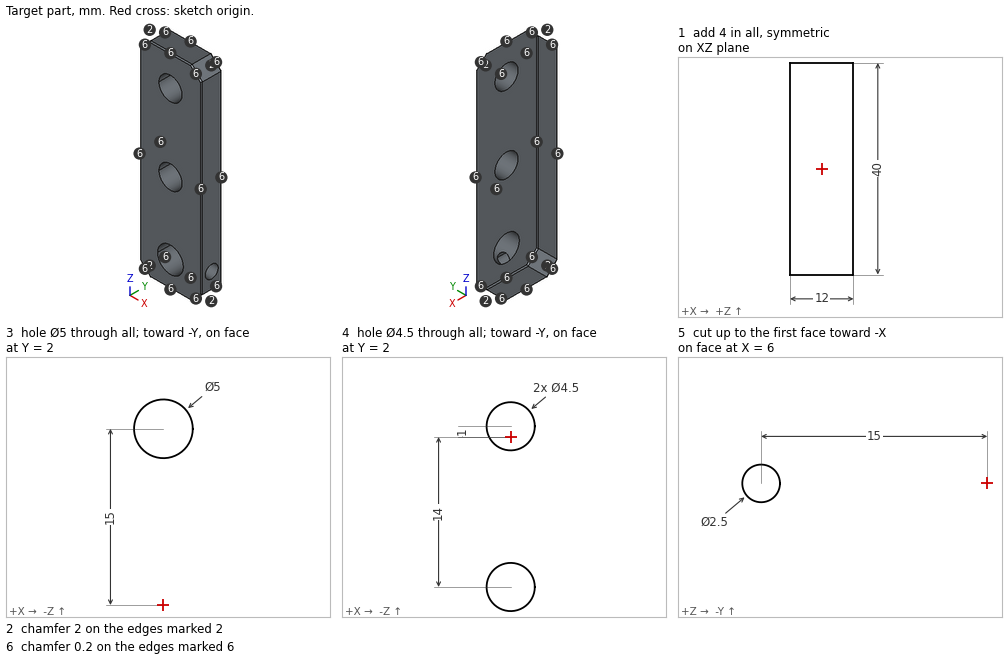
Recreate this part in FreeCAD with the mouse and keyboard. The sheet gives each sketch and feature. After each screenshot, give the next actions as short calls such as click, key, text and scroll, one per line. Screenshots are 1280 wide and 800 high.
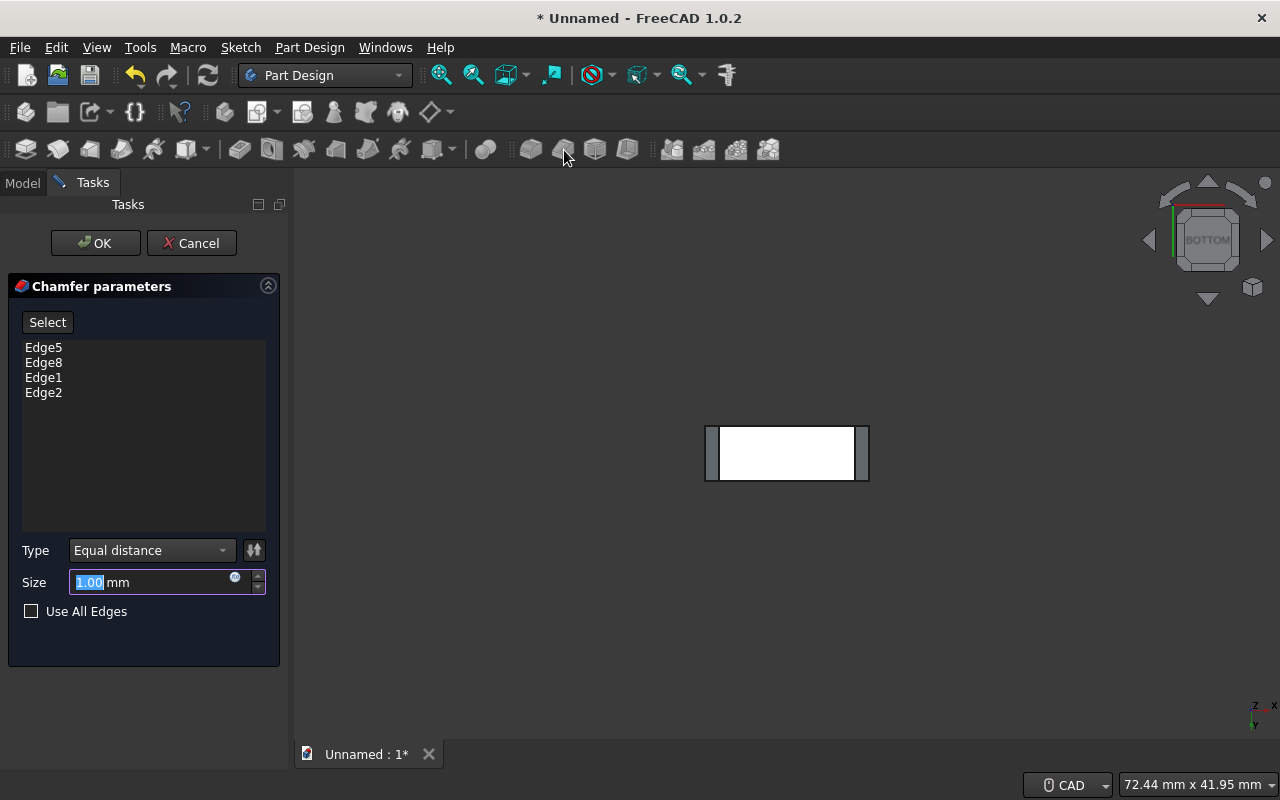
text(2)
key(Tab)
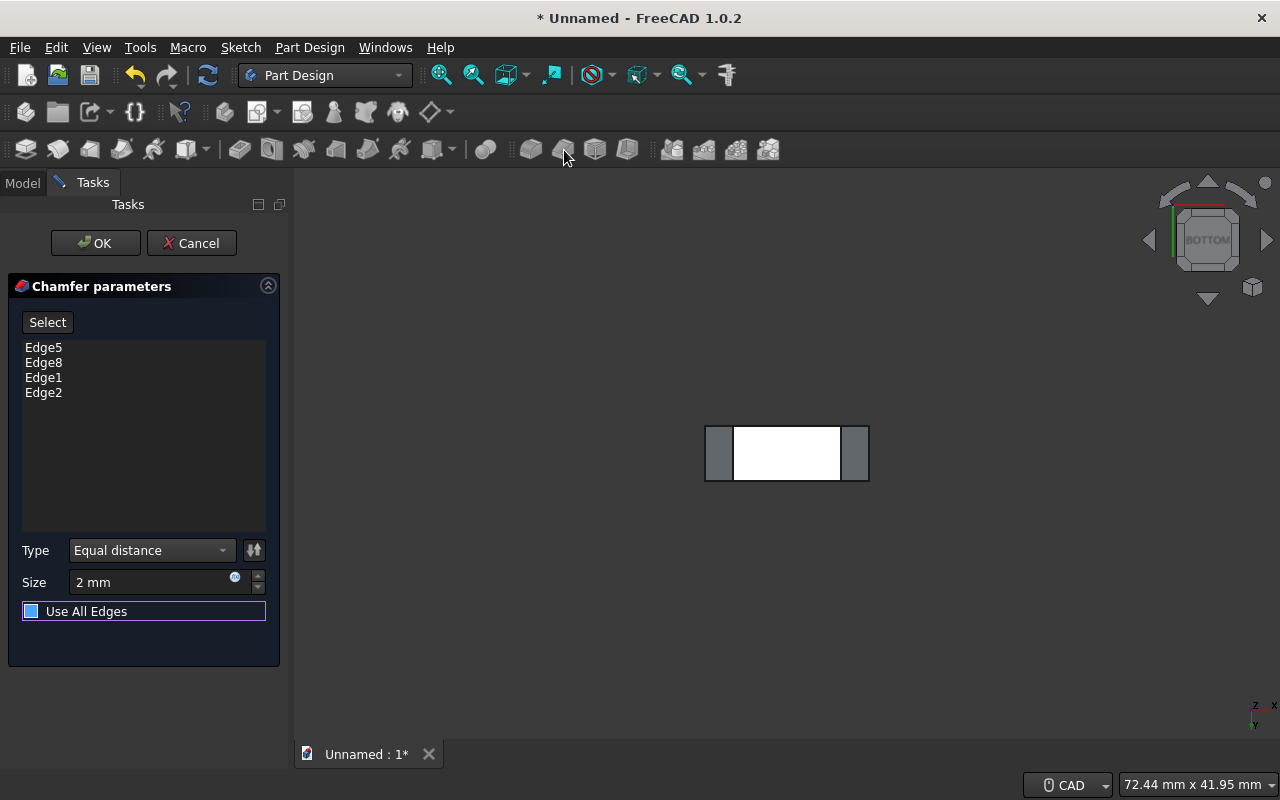
click(96, 243)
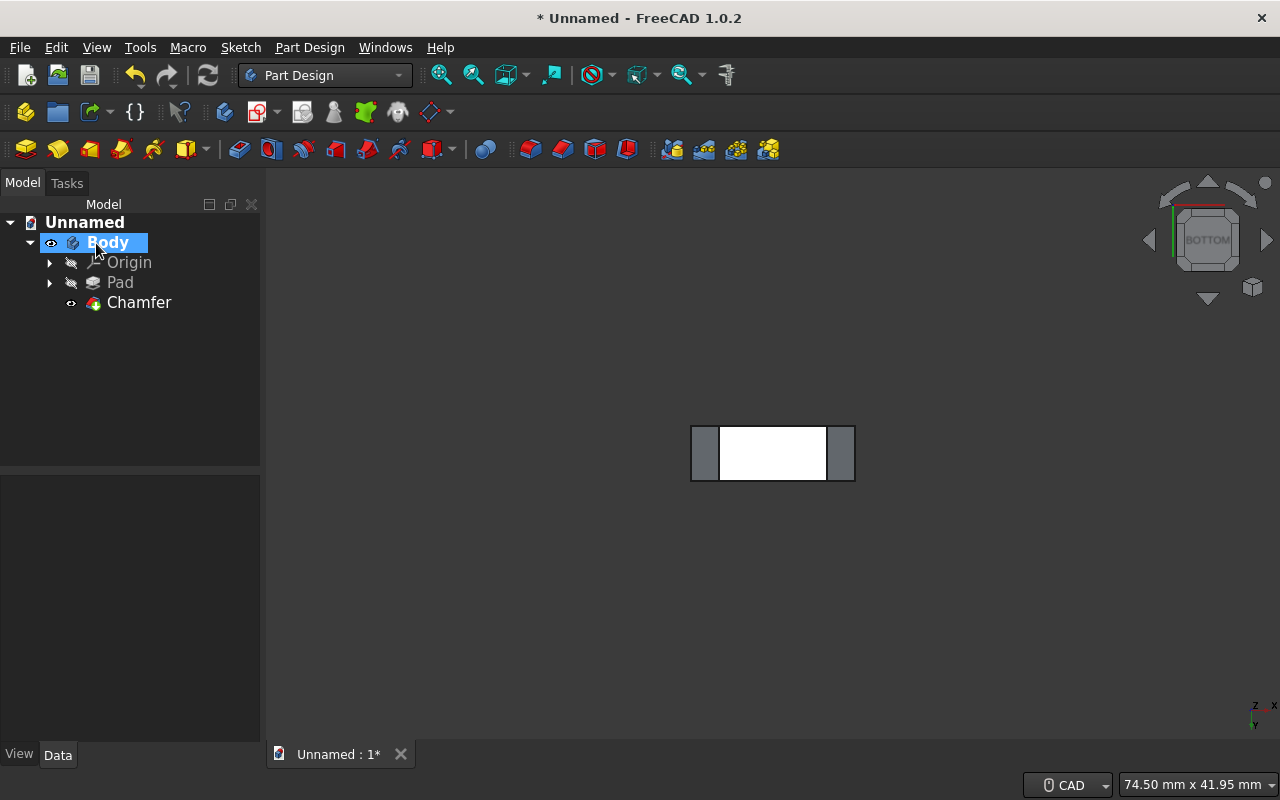
click(442, 76)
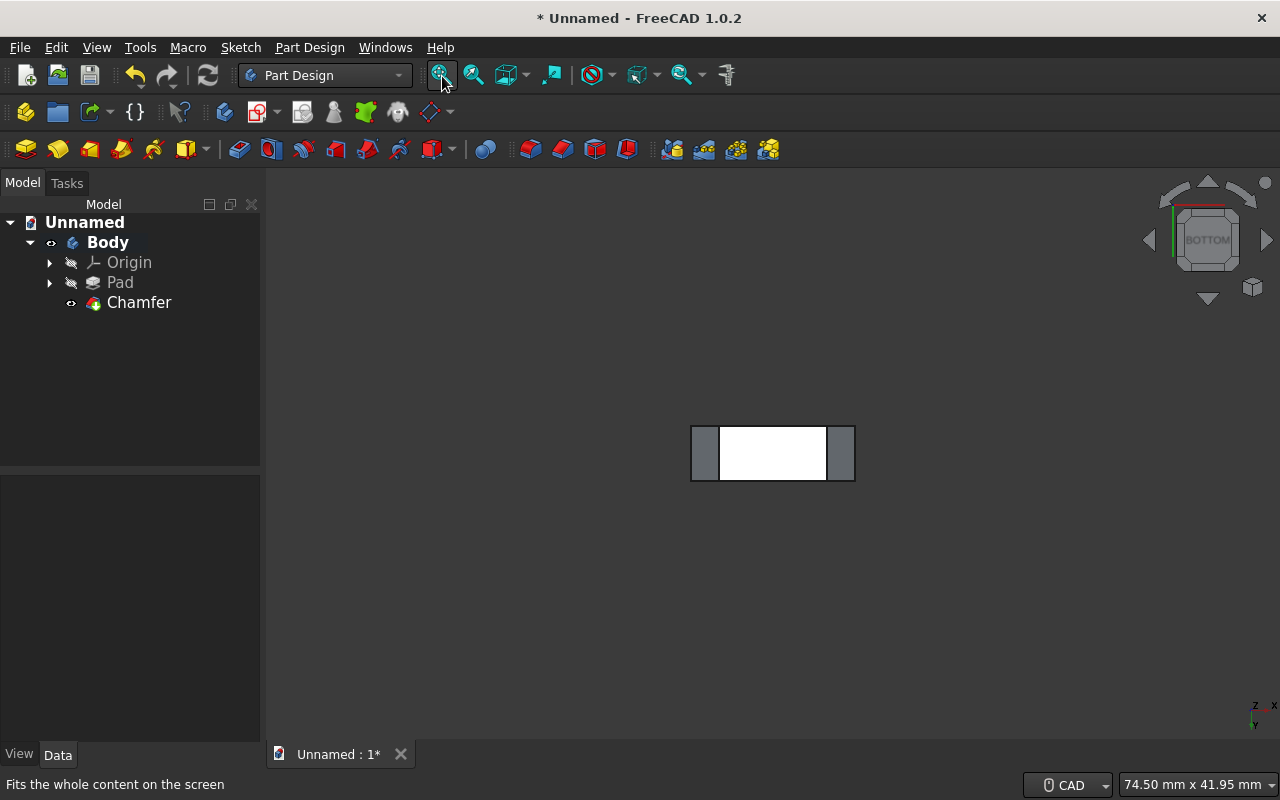
key(4)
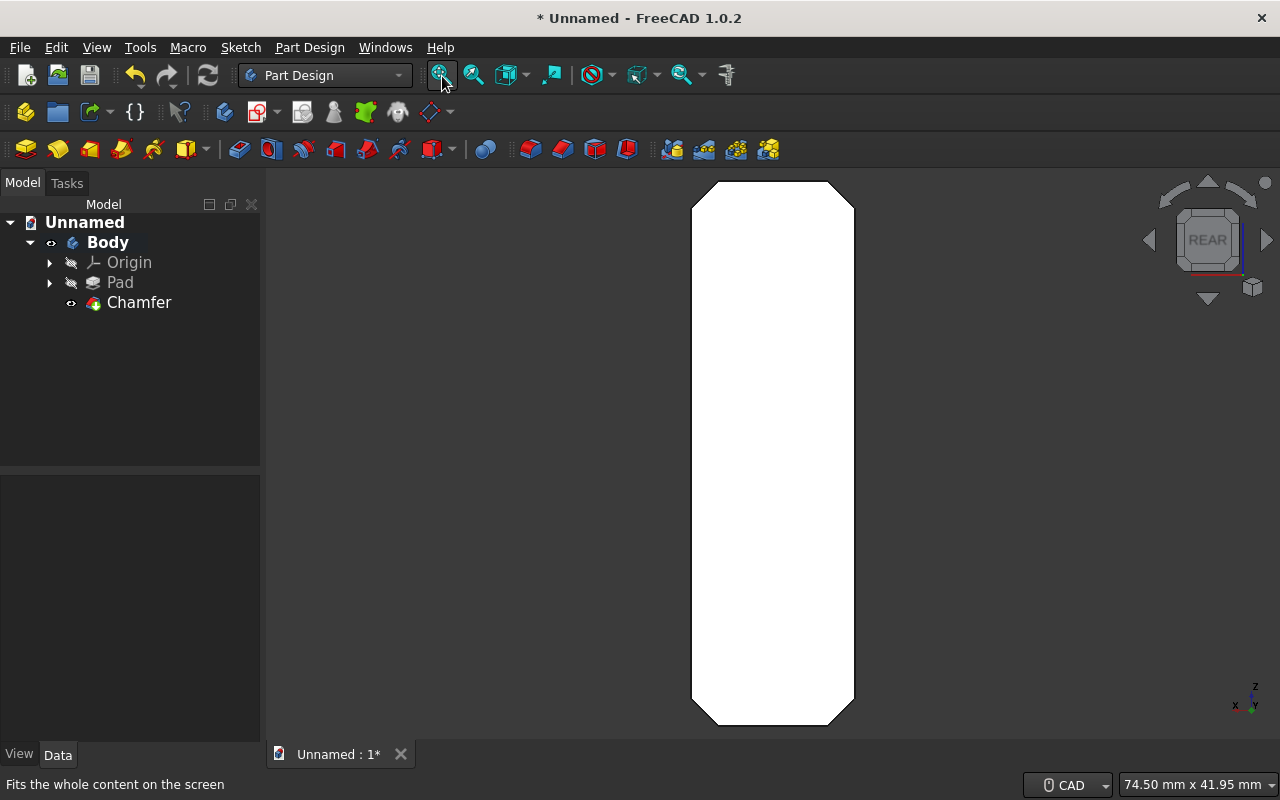
click(773, 297)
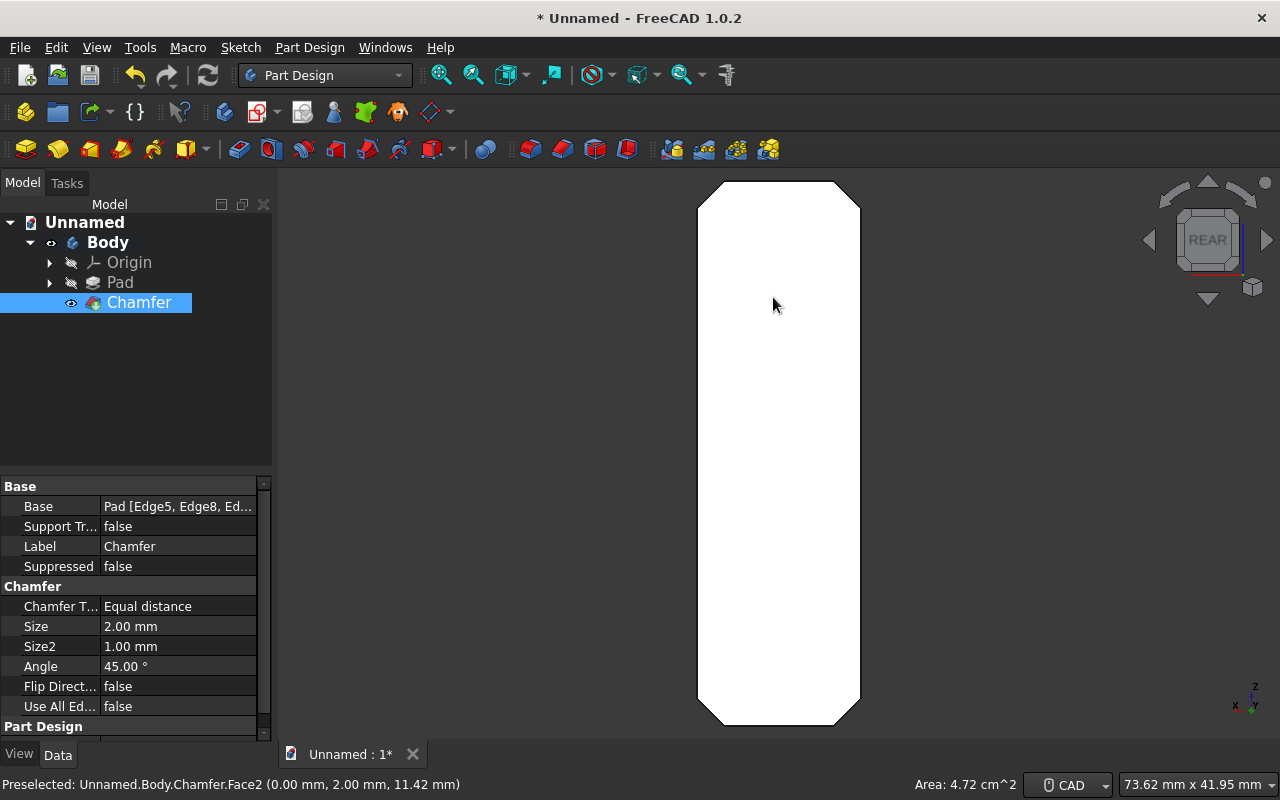
click(258, 112)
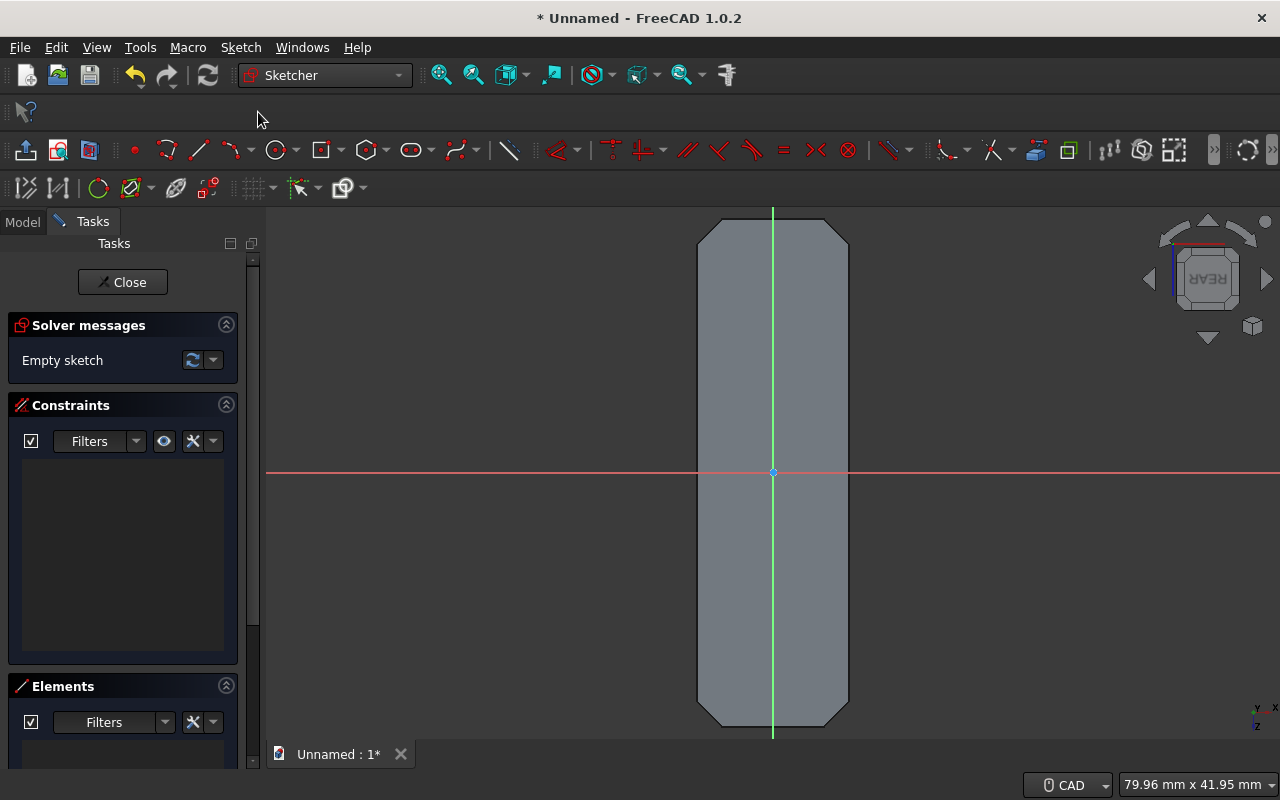
scroll(790, 235, up, 8)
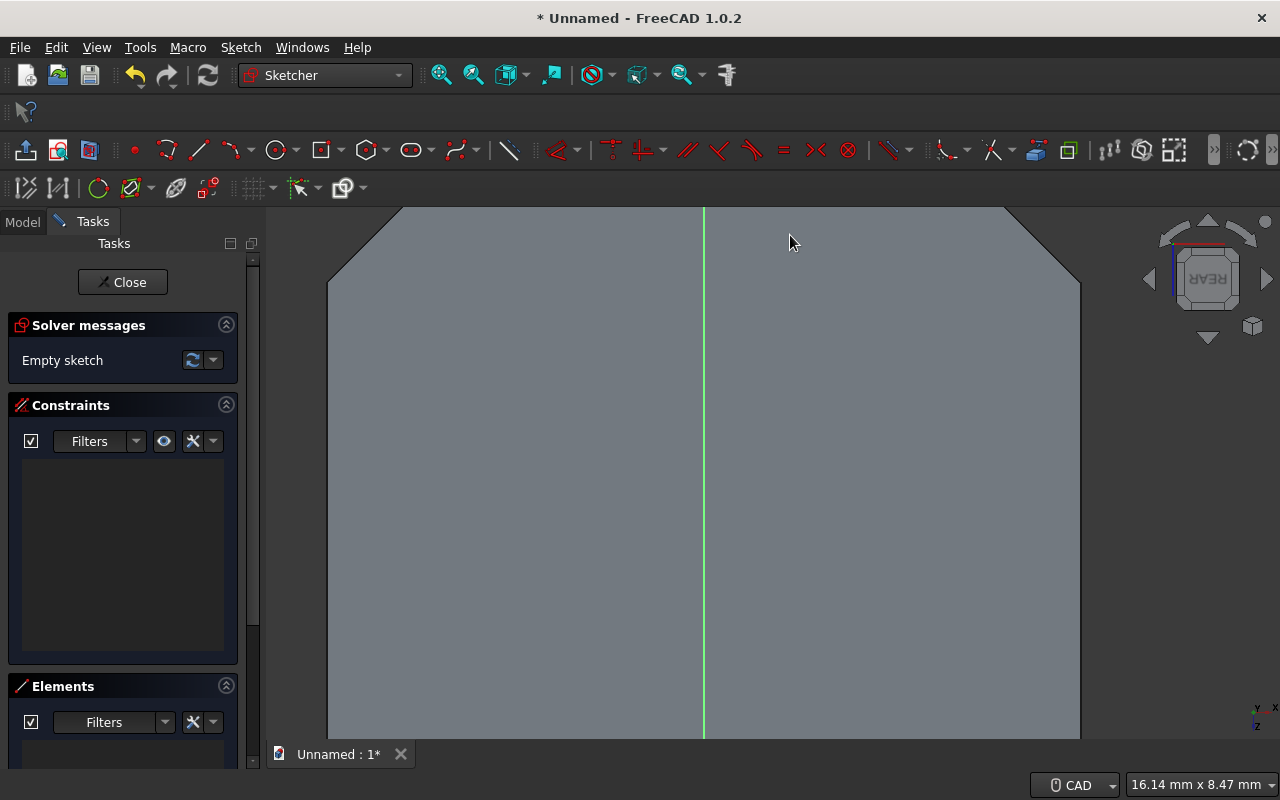
click(276, 150)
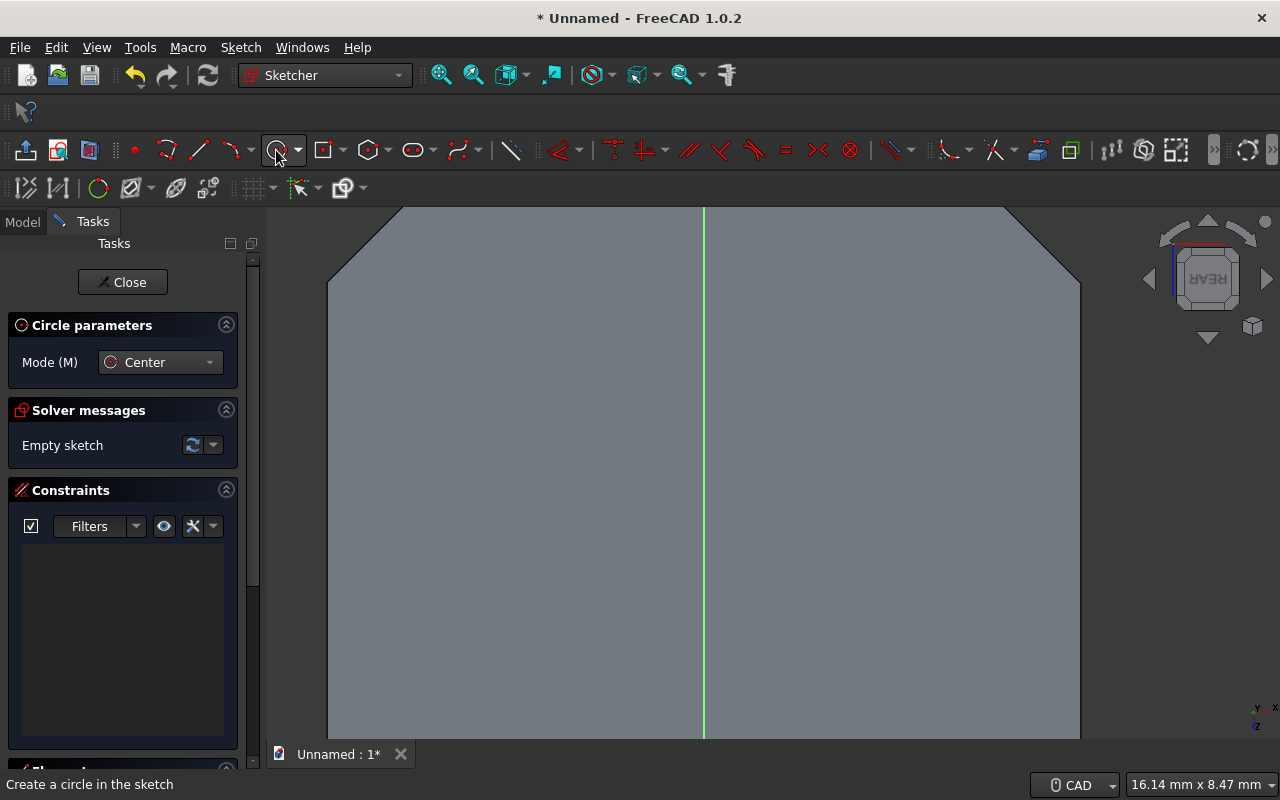
click(704, 471)
click(815, 360)
key(Escape)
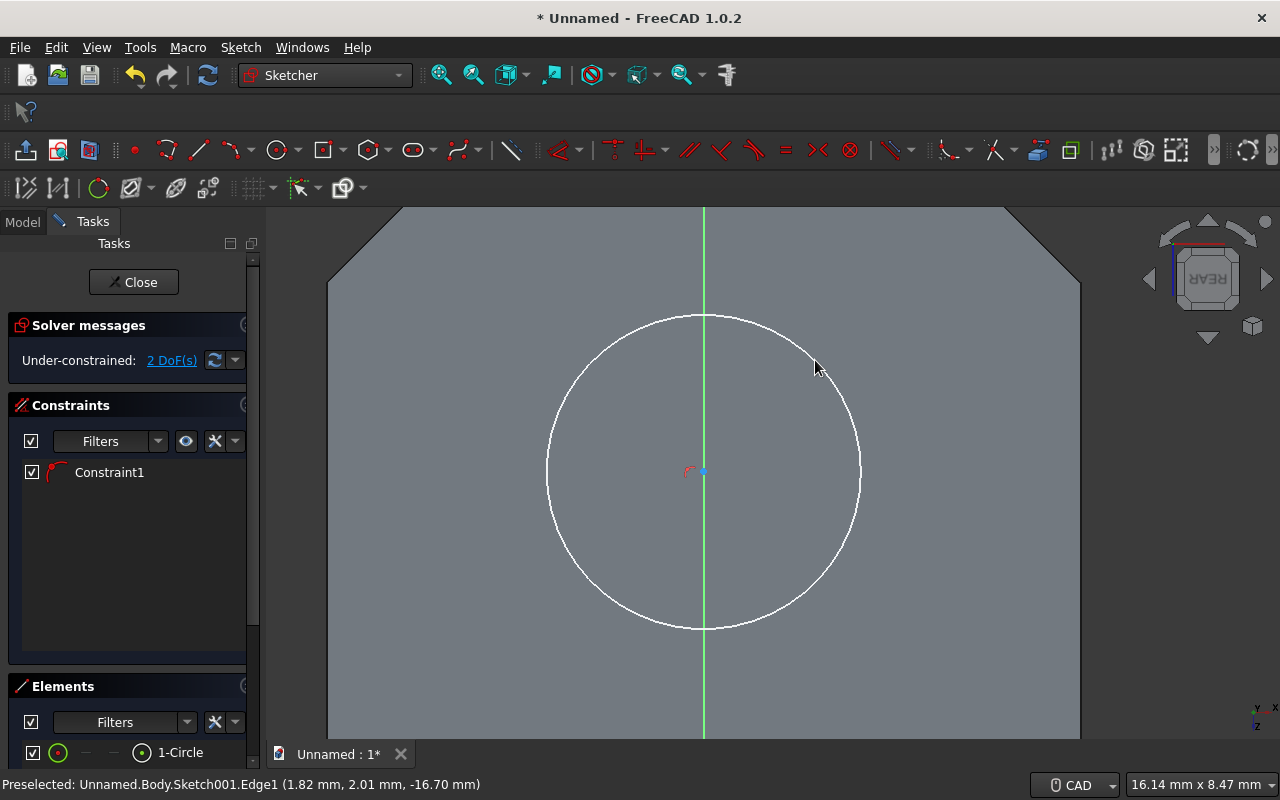
click(558, 150)